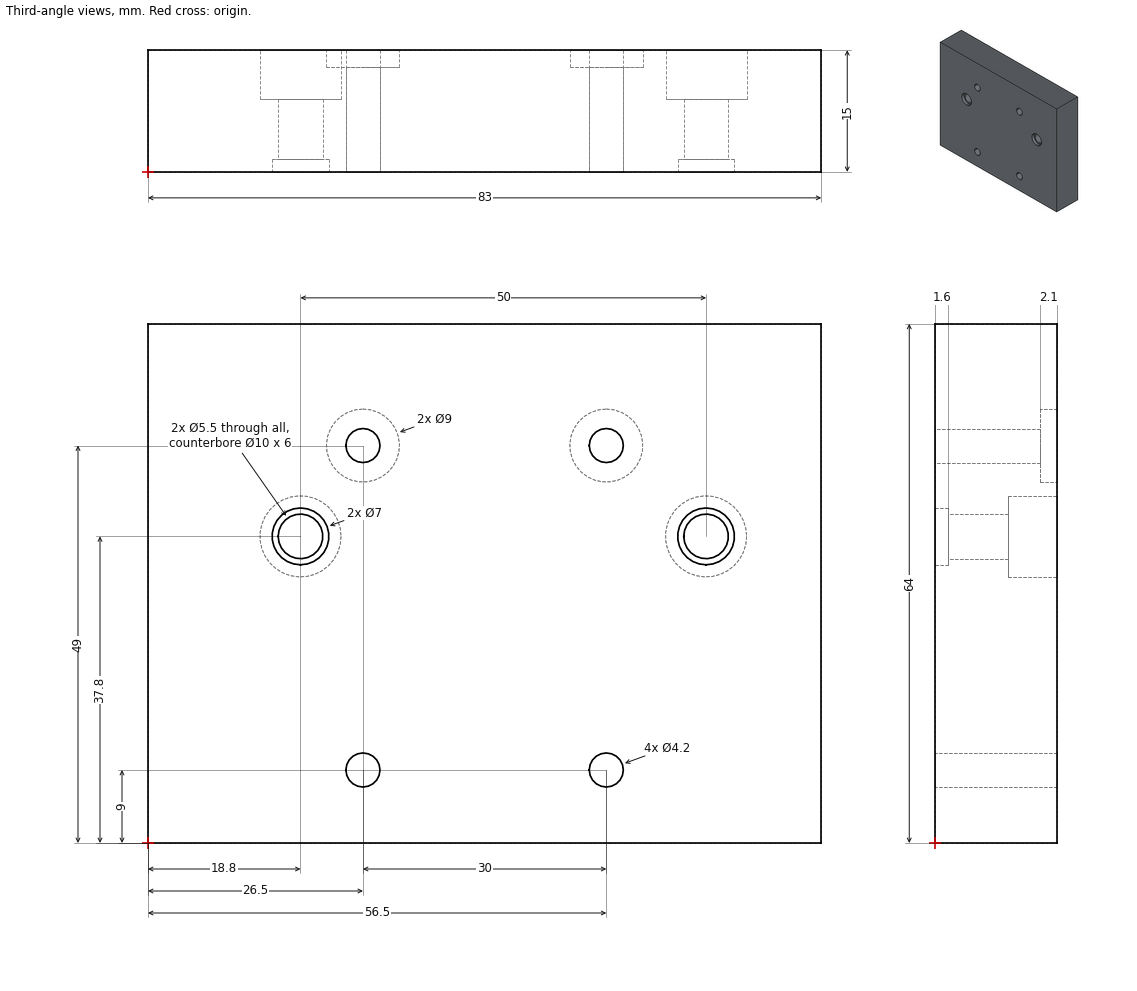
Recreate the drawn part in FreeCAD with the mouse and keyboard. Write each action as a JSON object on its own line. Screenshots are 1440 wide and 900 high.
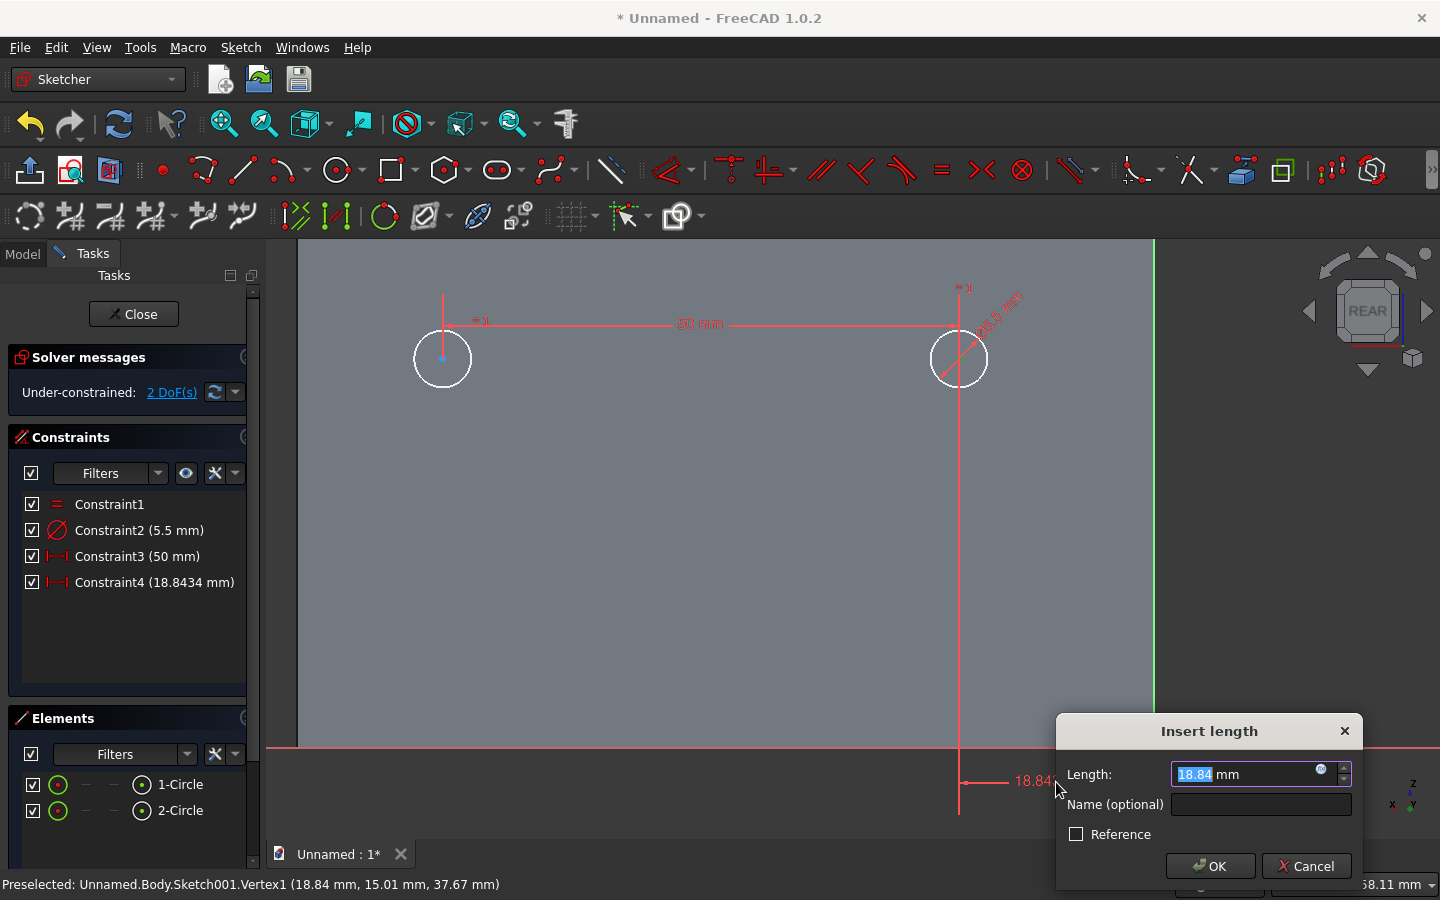
{"action": "type", "text": "18.8"}
{"action": "key", "text": "Return"}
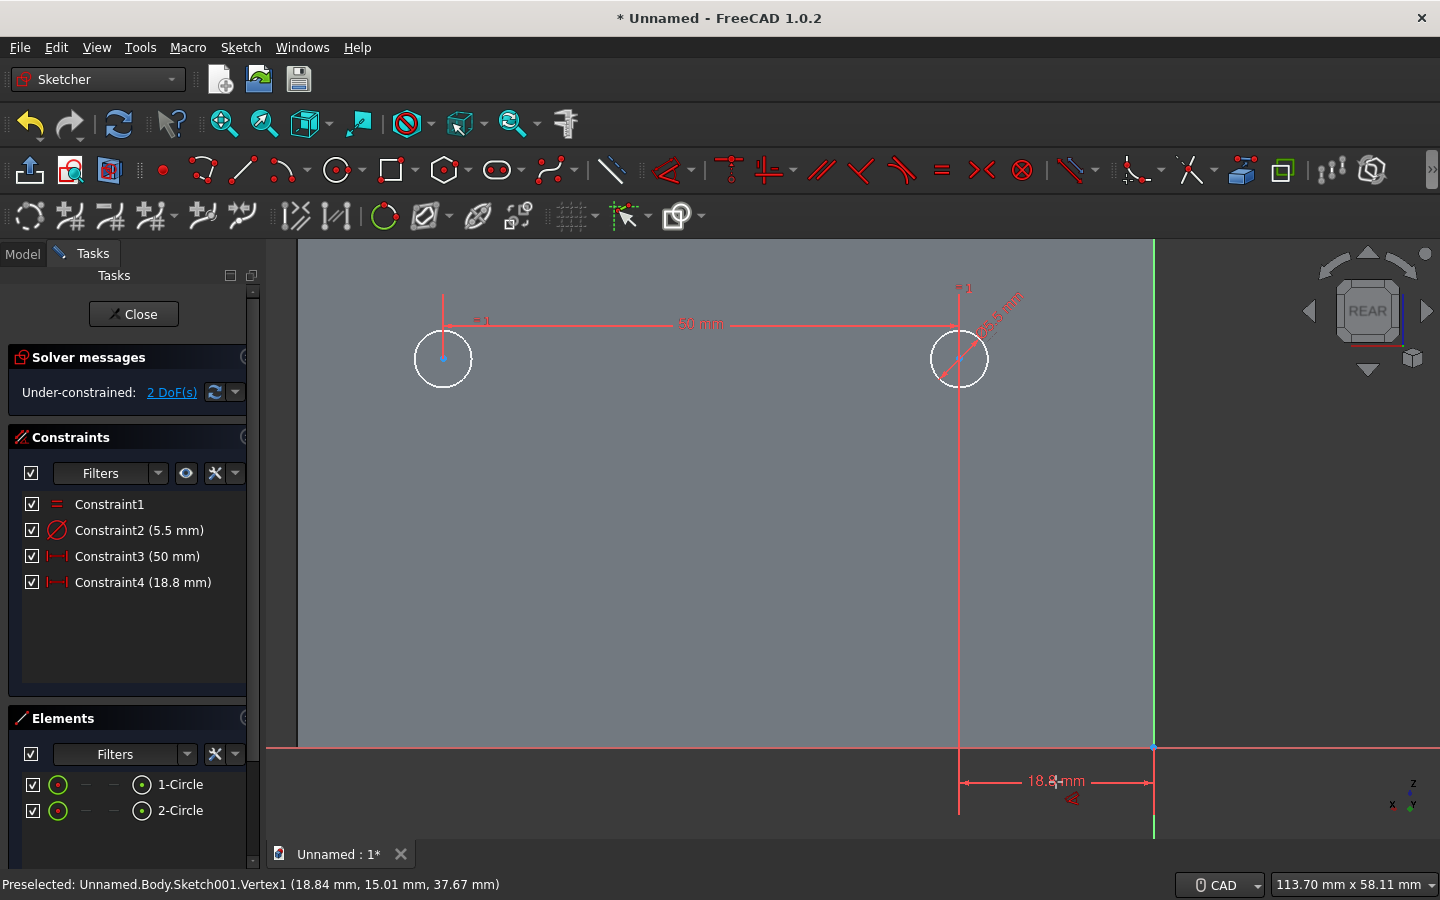
{"action": "left_click", "coordinate": [959, 359]}
{"action": "left_click", "coordinate": [1188, 553]}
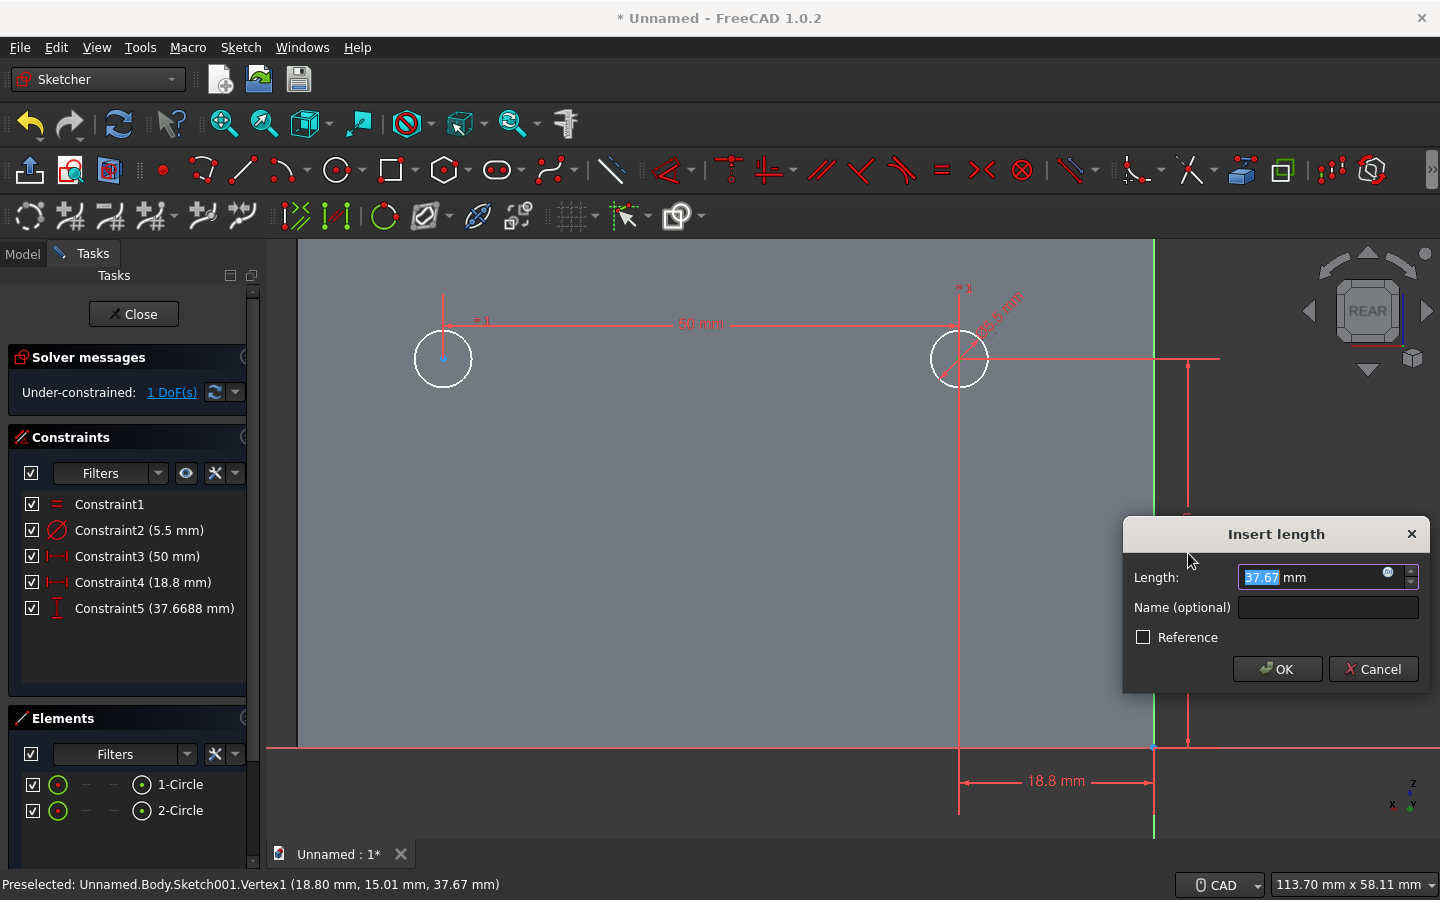
{"action": "type", "text": "37.8"}
{"action": "key", "text": "Return"}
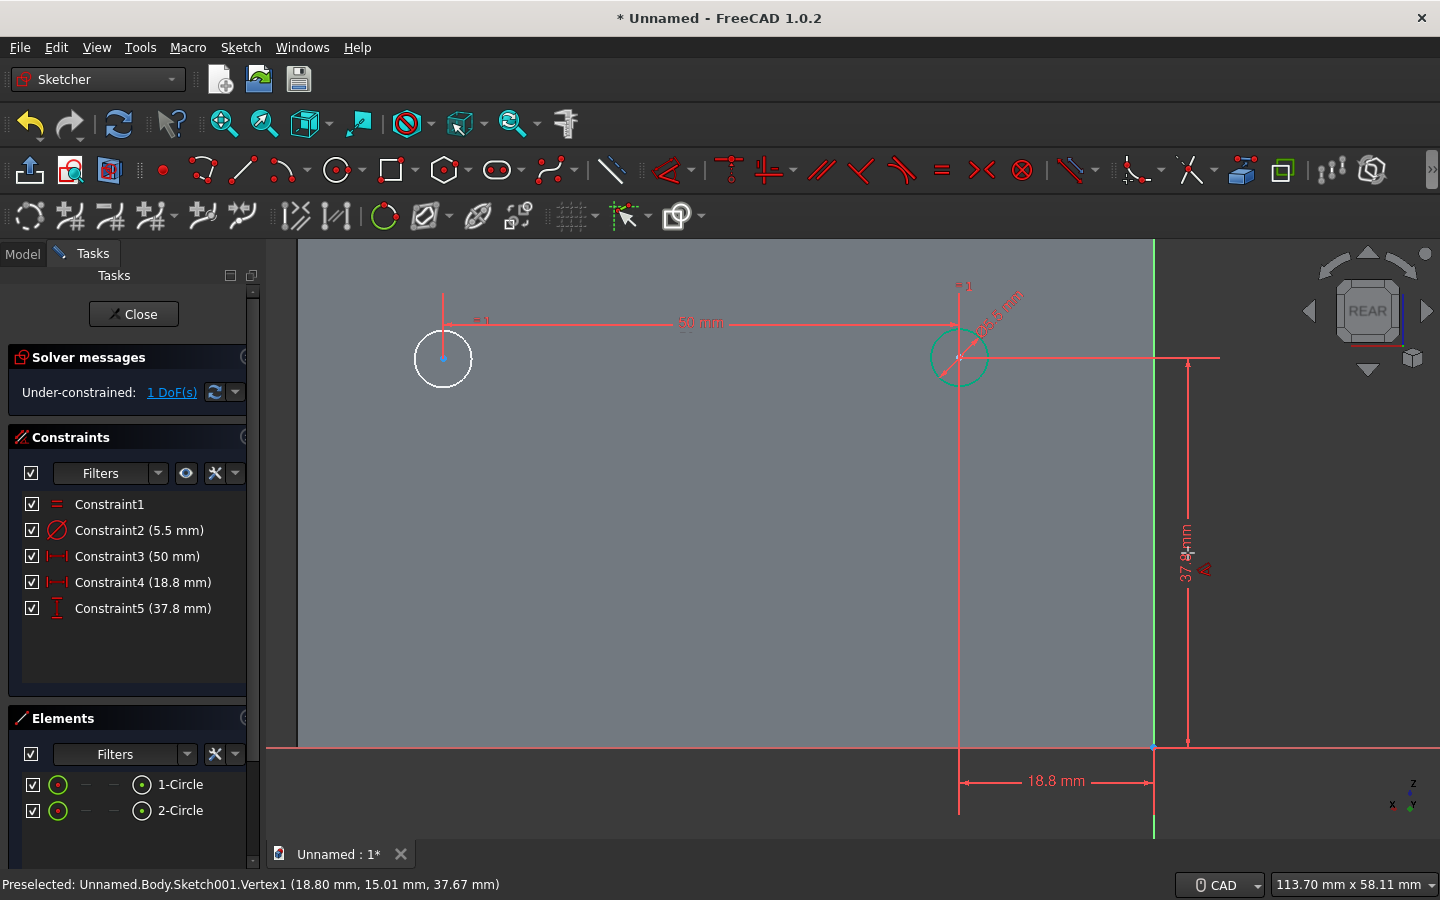
{"action": "left_click", "coordinate": [443, 359]}
{"action": "left_click", "coordinate": [1188, 464]}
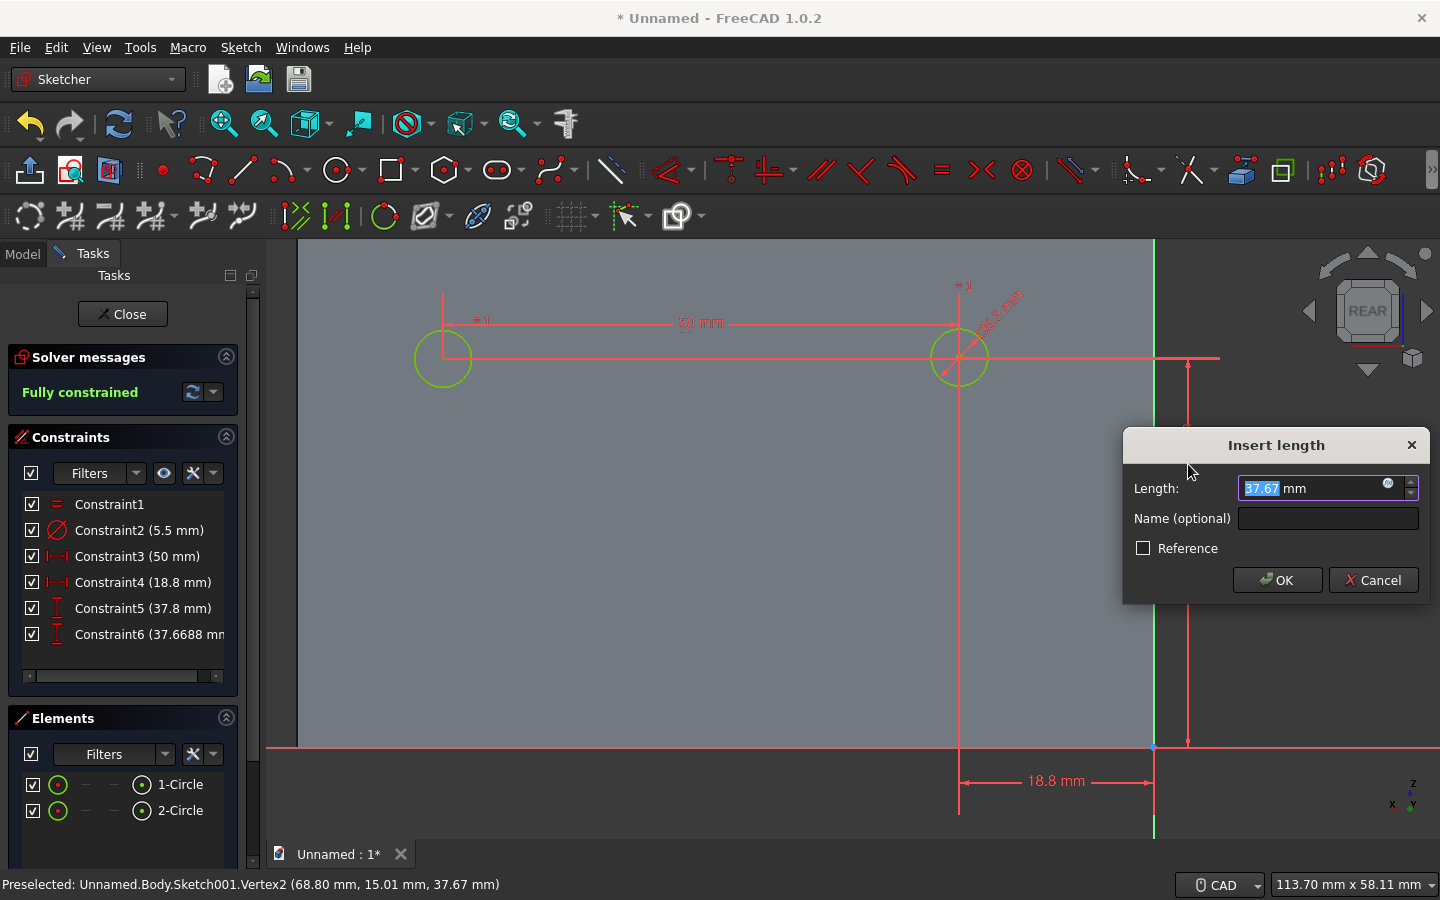
{"action": "type", "text": "37.8"}
{"action": "key", "text": "Return"}
{"action": "key", "text": "Escape"}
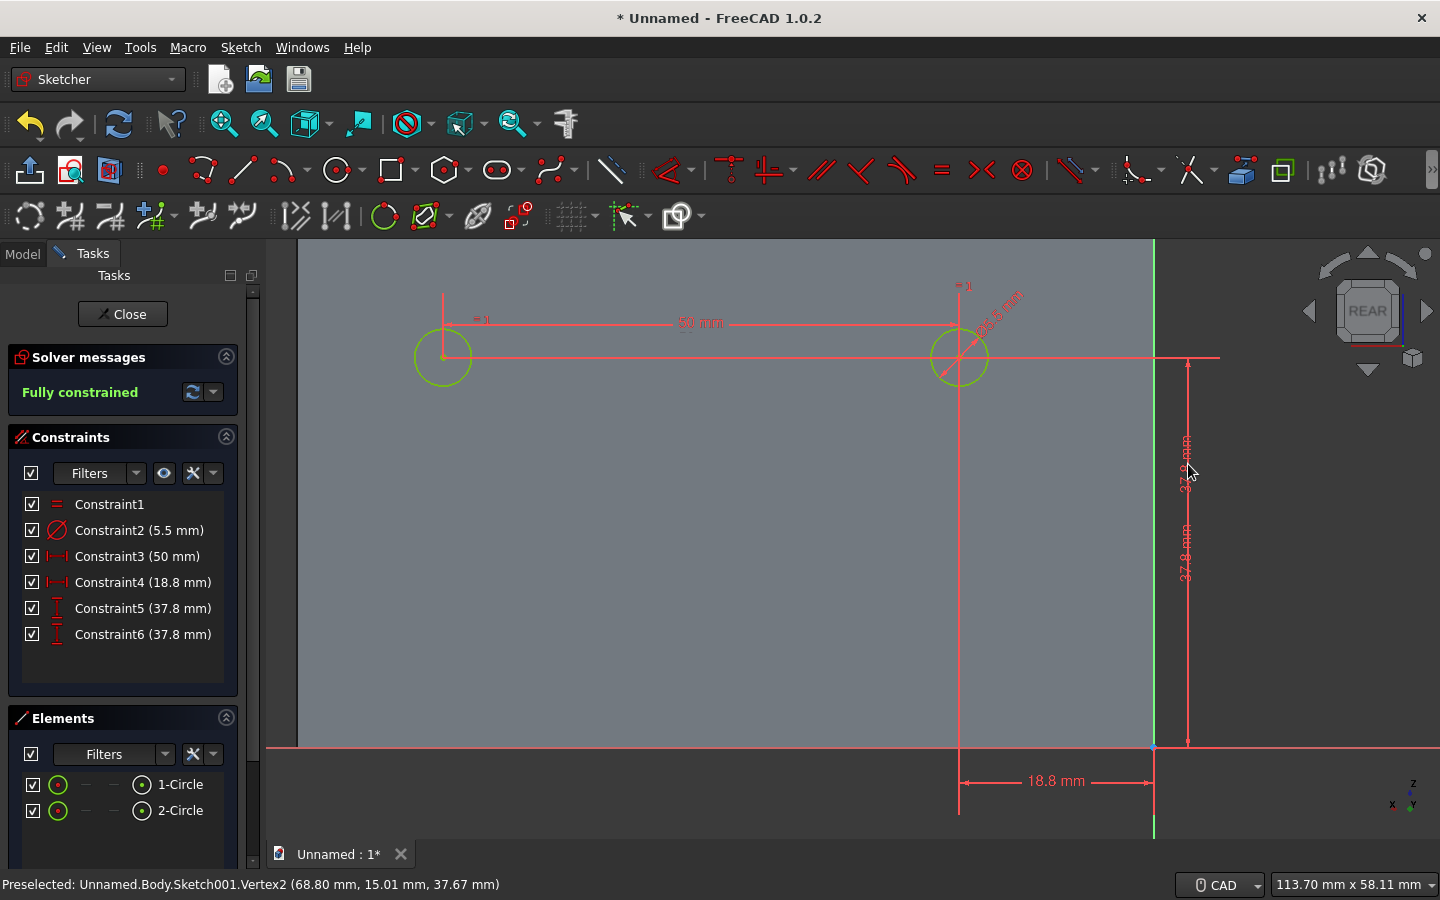
{"action": "left_click", "coordinate": [123, 314]}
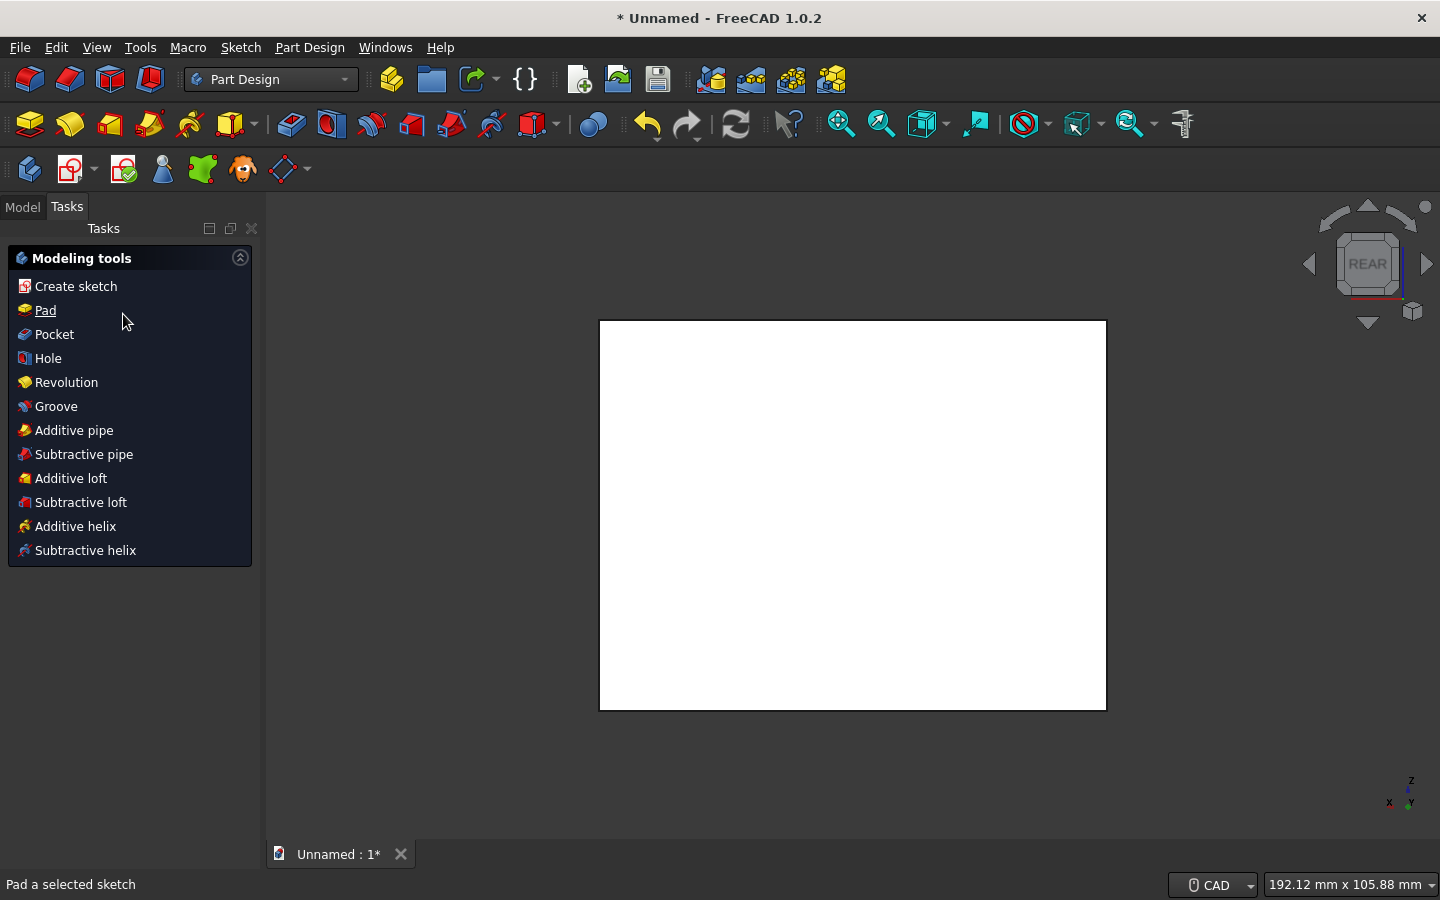
{"action": "left_click", "coordinate": [332, 124]}